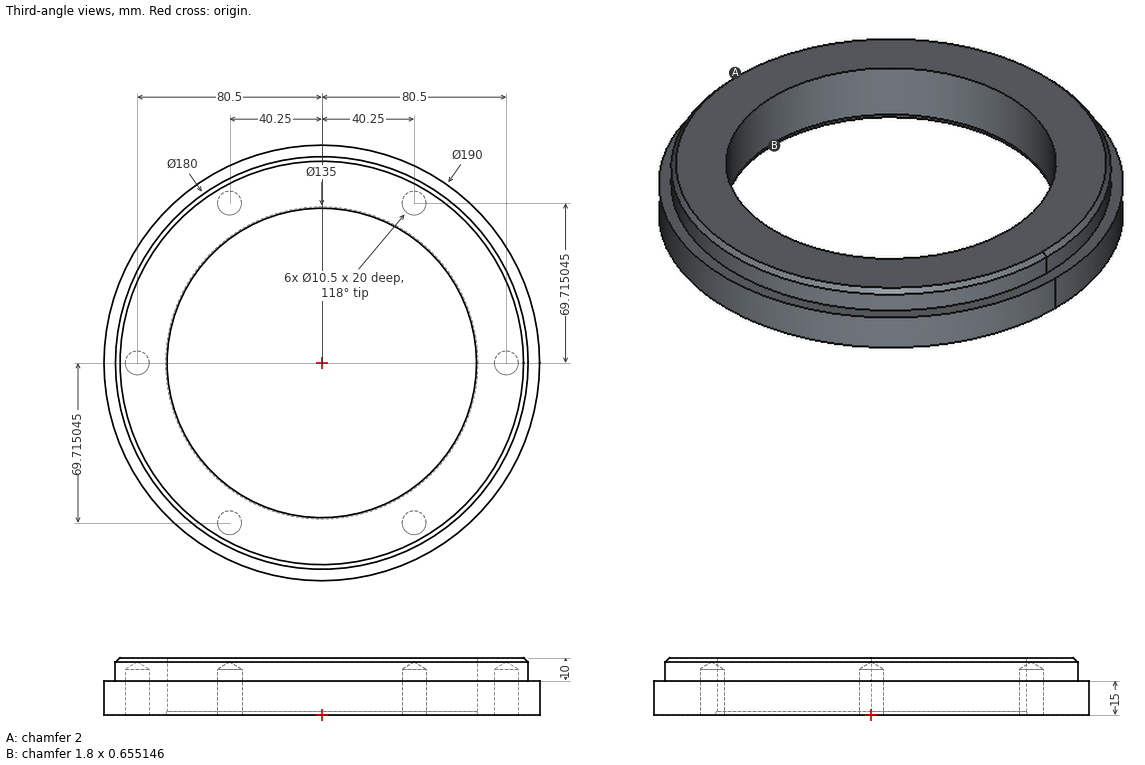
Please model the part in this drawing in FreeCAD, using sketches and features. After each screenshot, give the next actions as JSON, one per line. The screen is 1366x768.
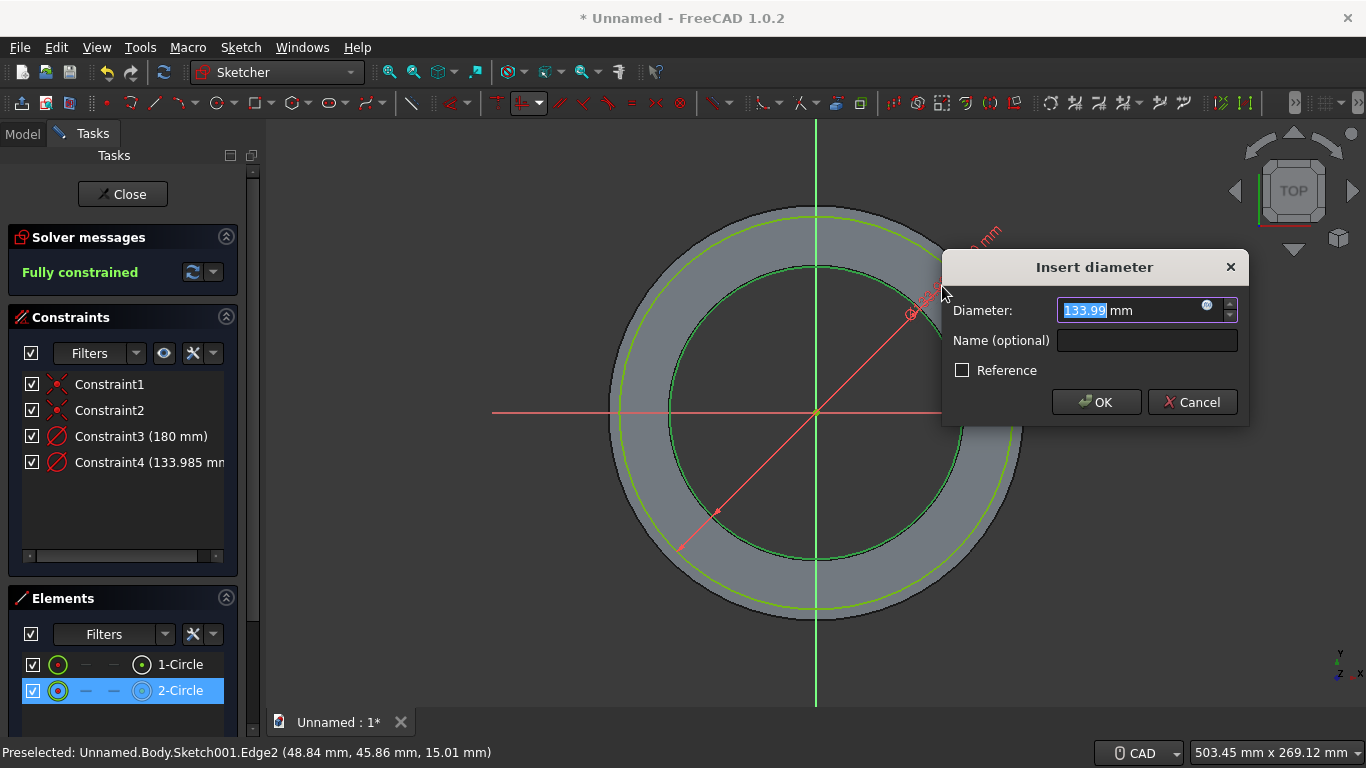
{"action": "type", "text": "135"}
{"action": "key", "text": "Return"}
{"action": "key", "text": "Escape"}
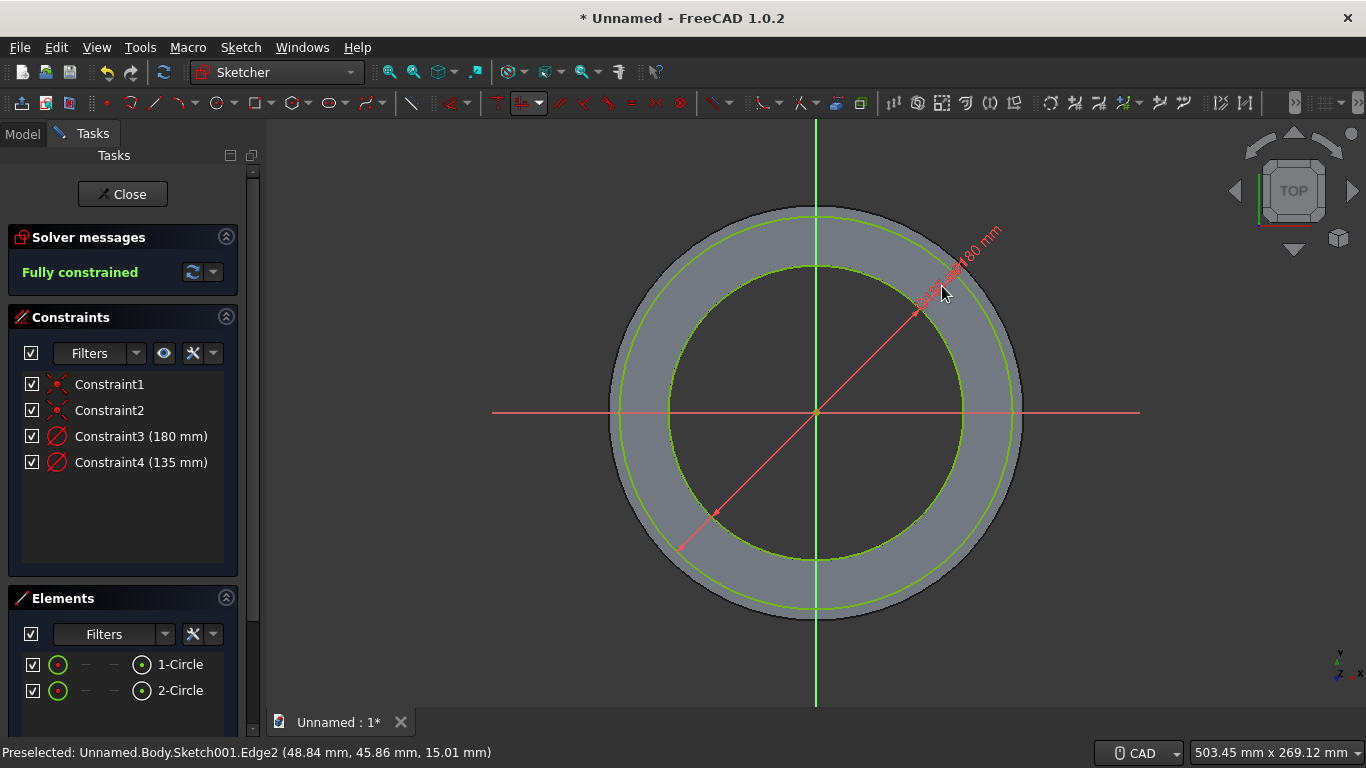
{"action": "left_click", "coordinate": [123, 194]}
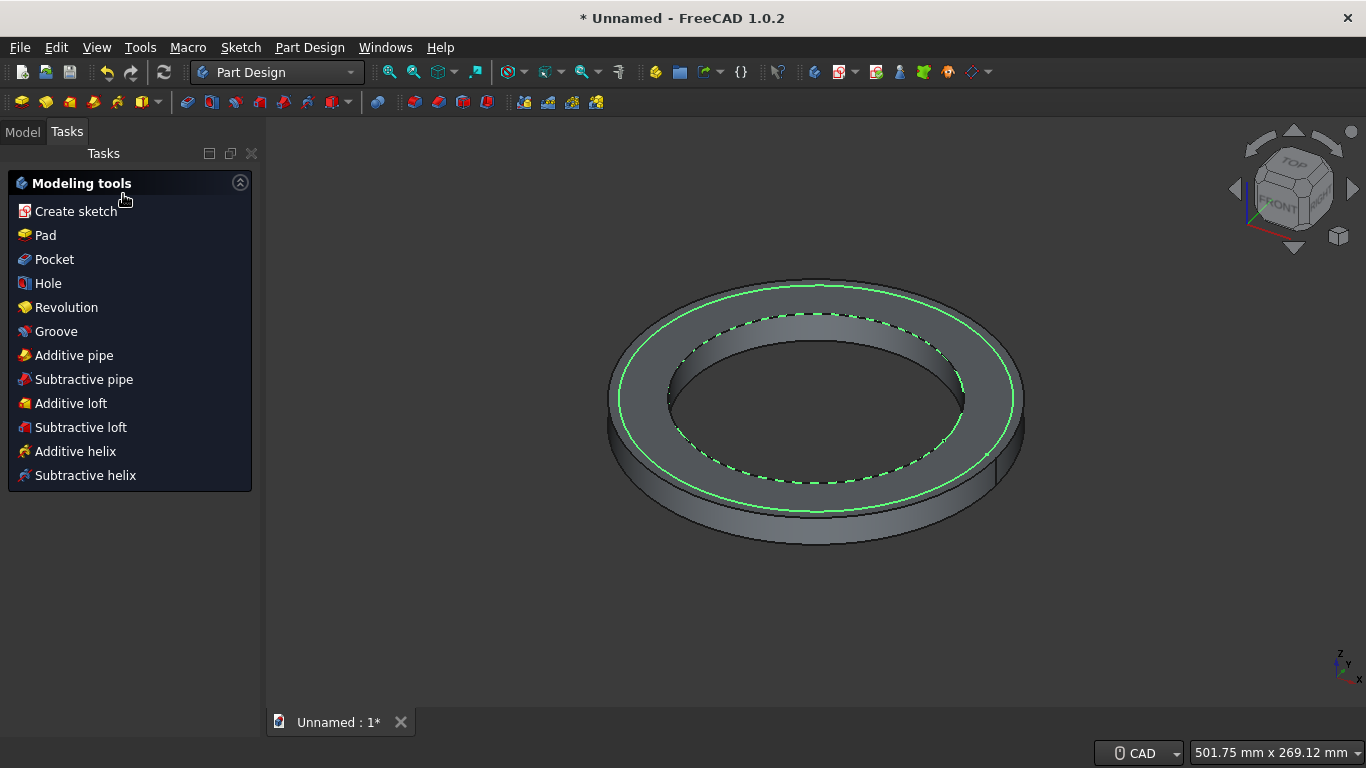
{"action": "left_click", "coordinate": [22, 102]}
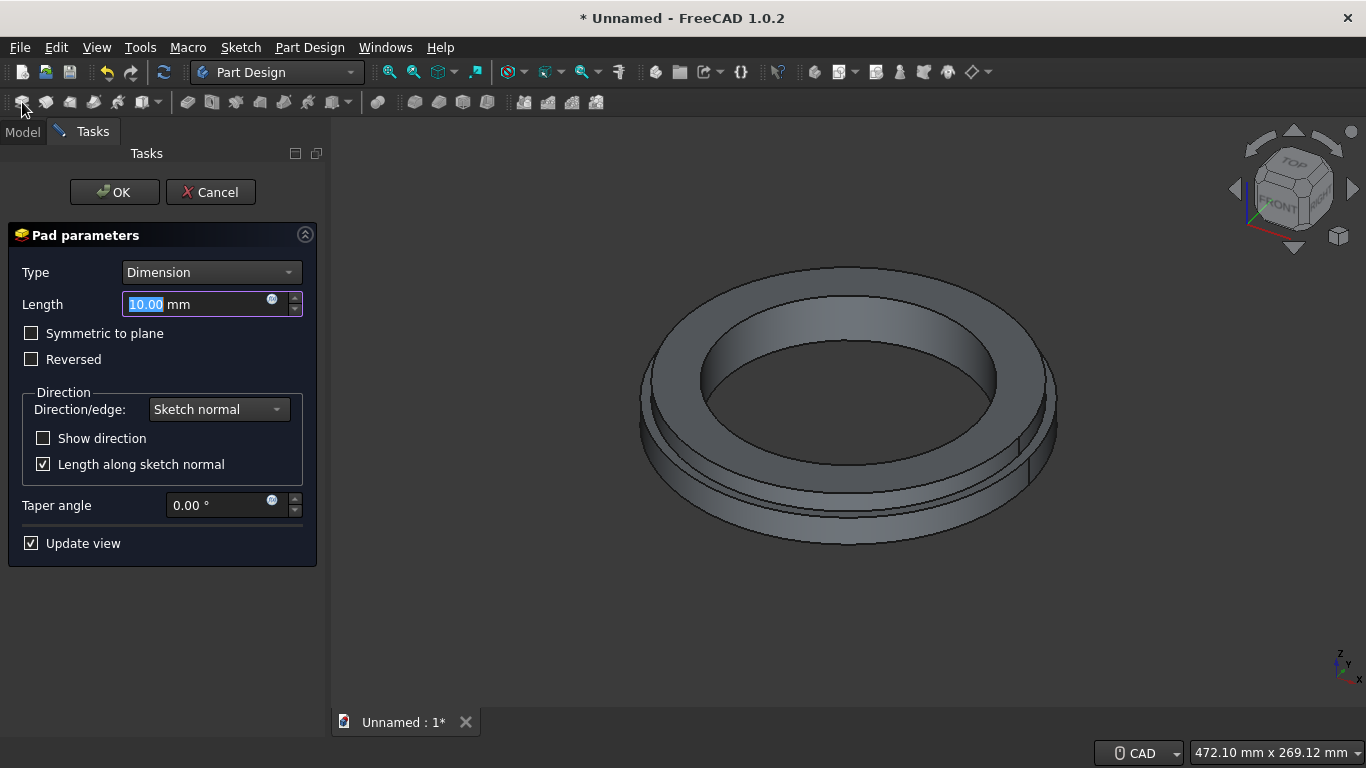
{"action": "type", "text": "10"}
{"action": "key", "text": "Tab"}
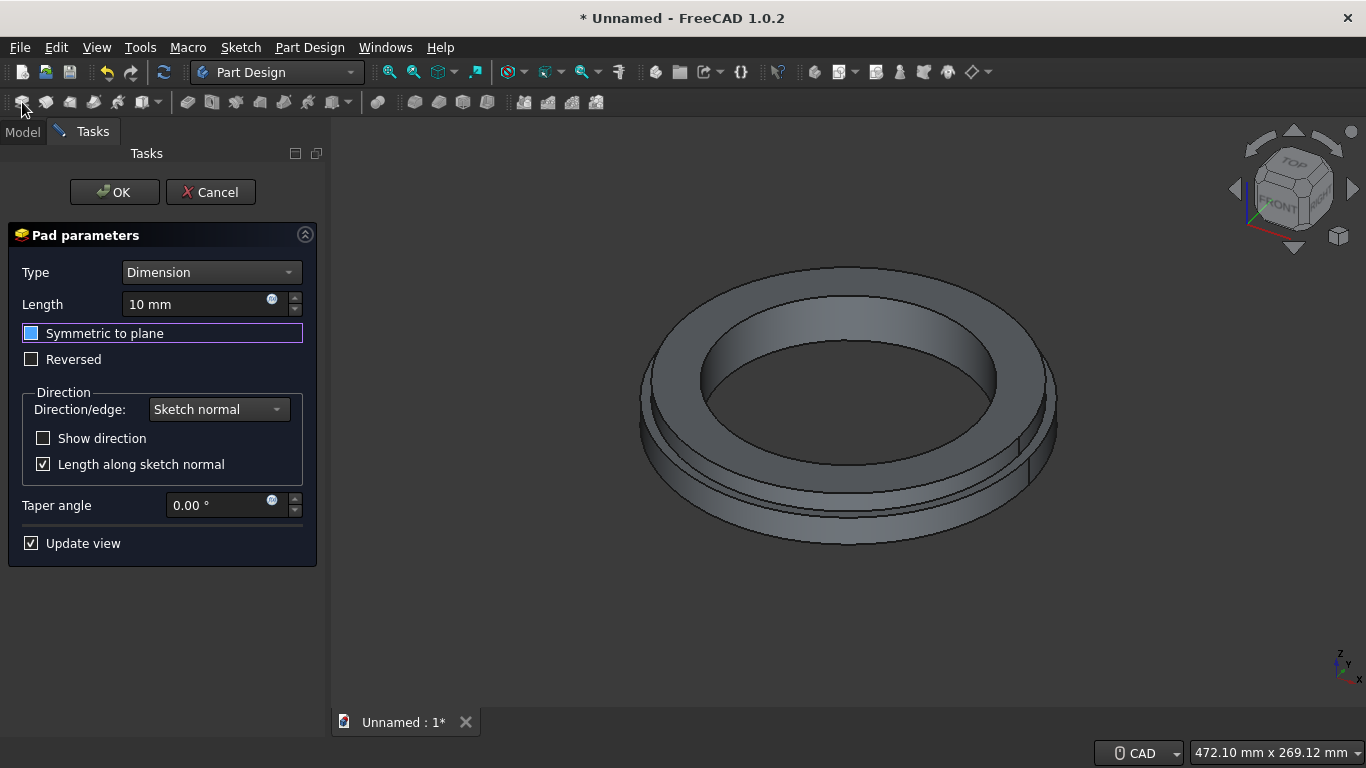
{"action": "left_click", "coordinate": [115, 192]}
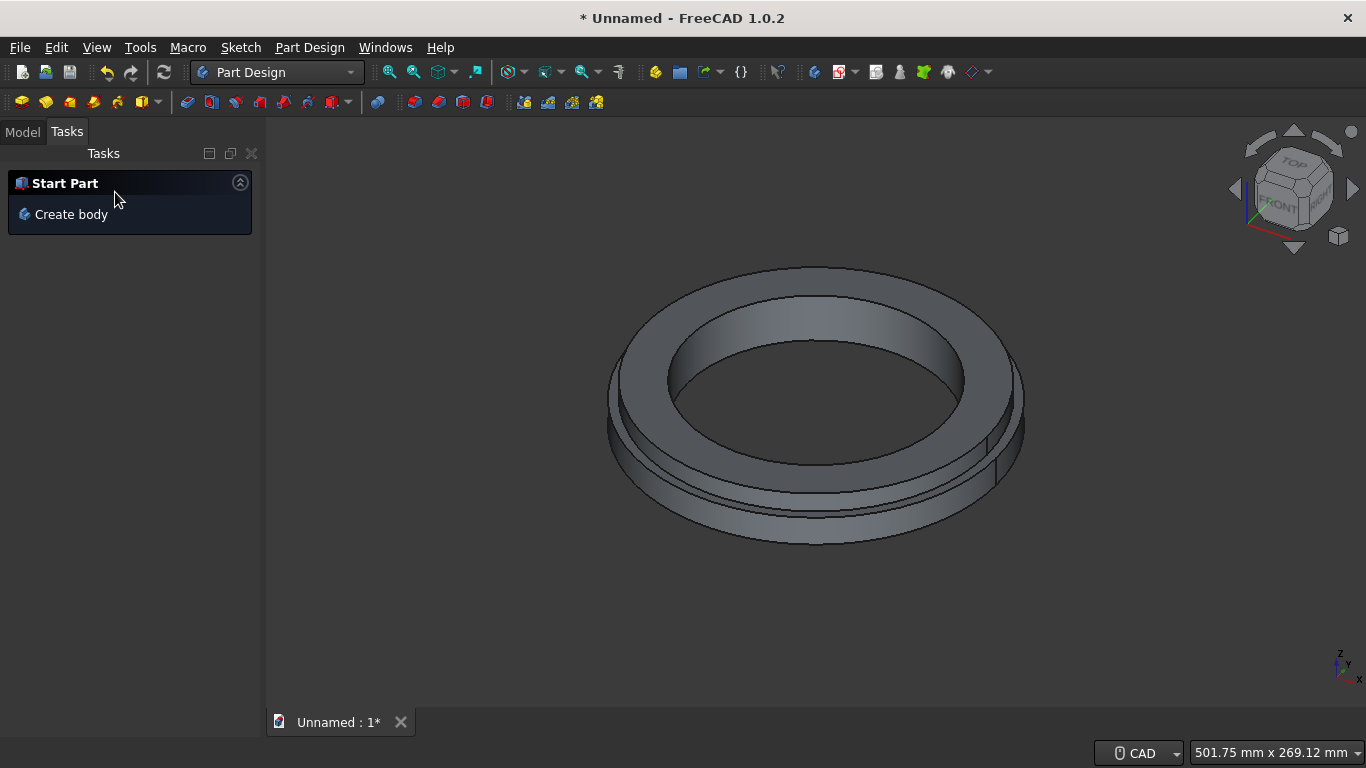
{"action": "left_click", "coordinate": [620, 391]}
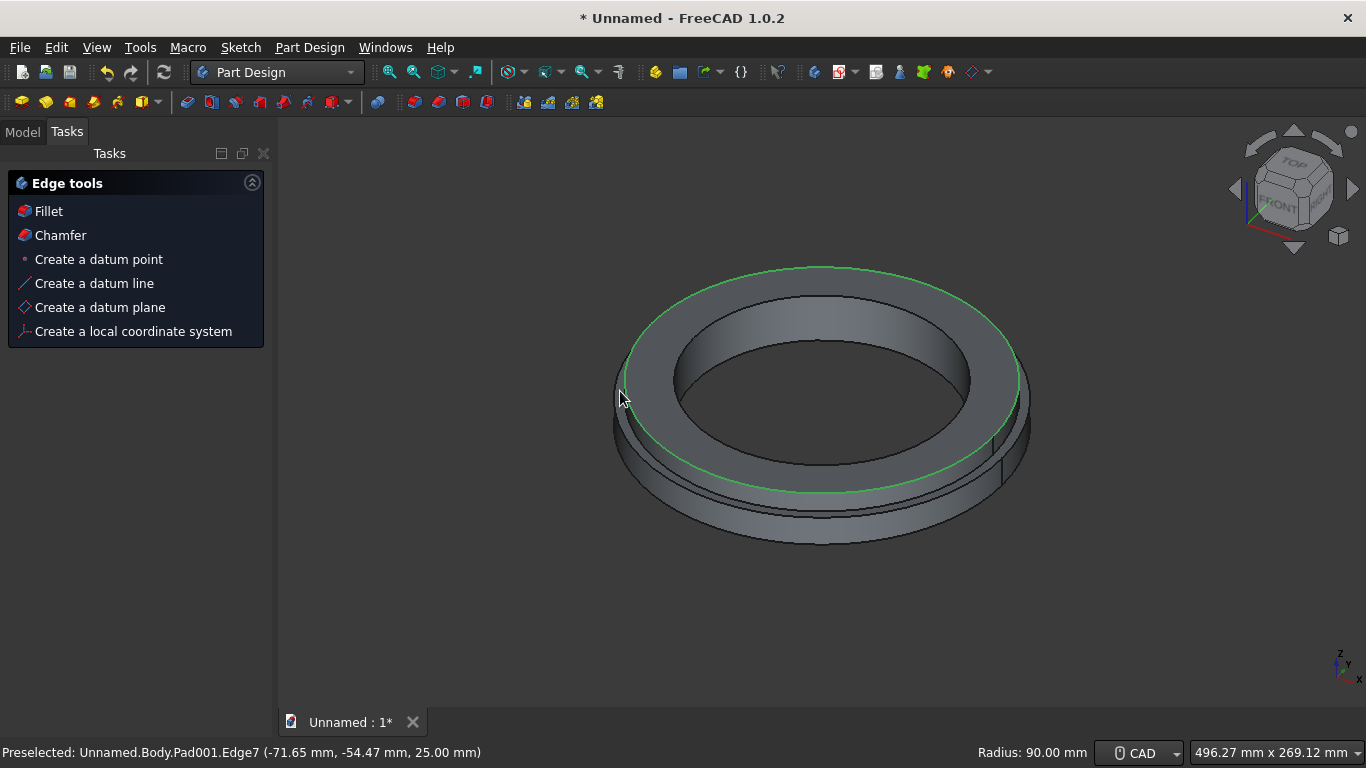
{"action": "left_click", "coordinate": [440, 102]}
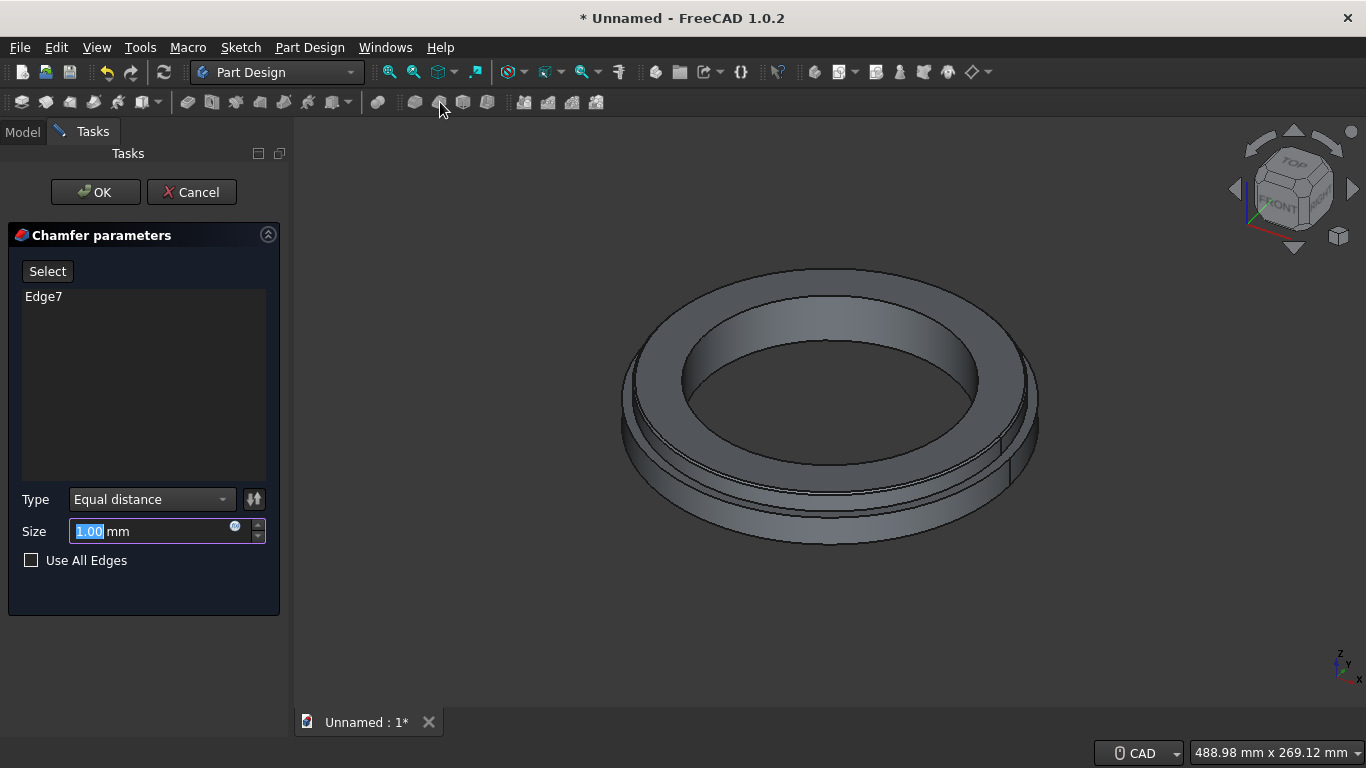
{"action": "type", "text": "2"}
{"action": "key", "text": "Tab"}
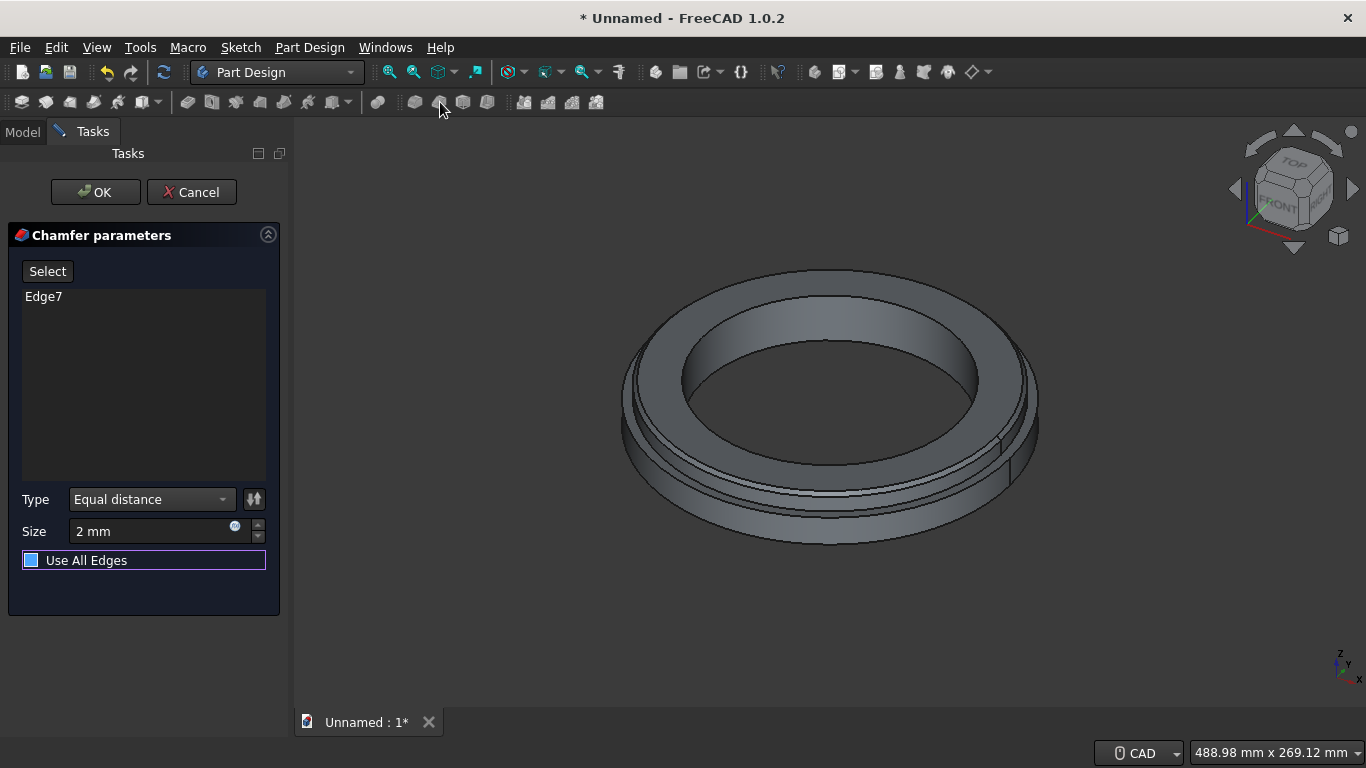
{"action": "left_click", "coordinate": [96, 192]}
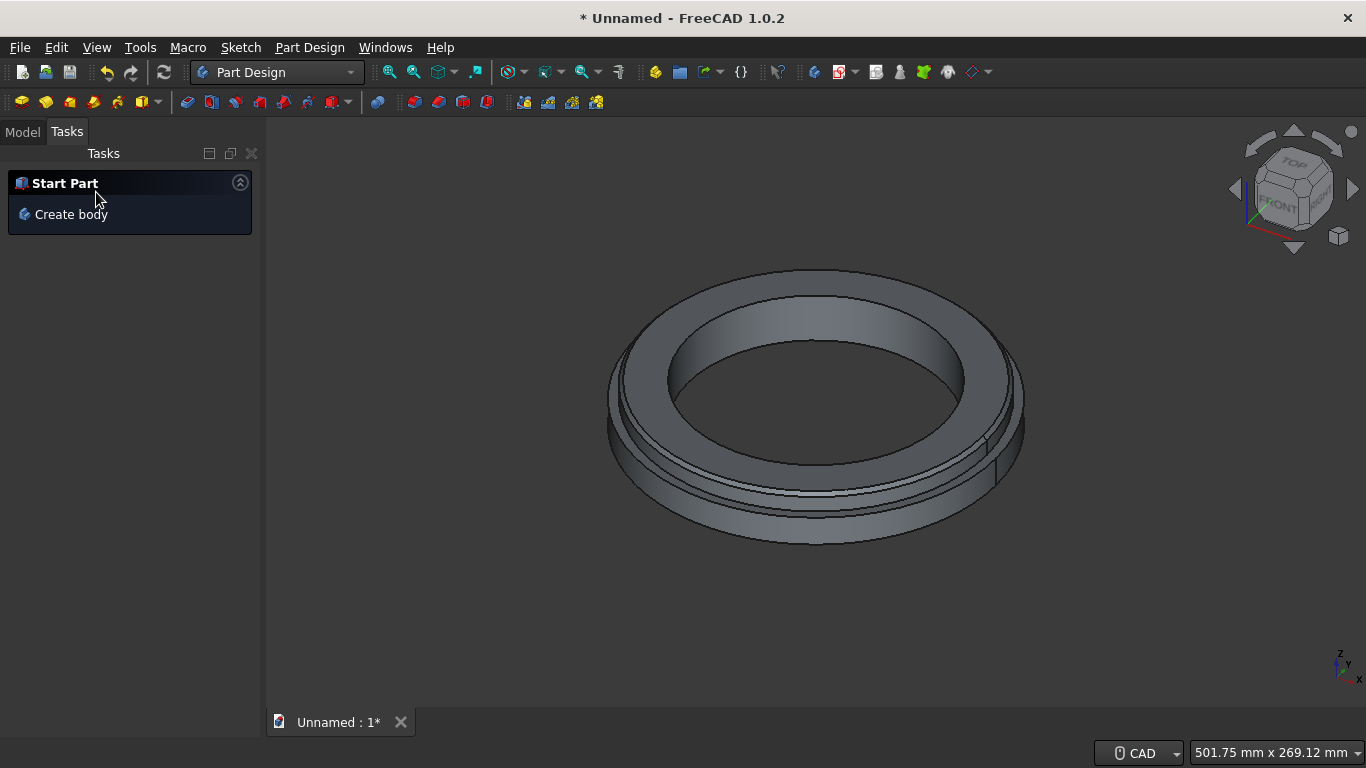
{"action": "key", "text": "0"}